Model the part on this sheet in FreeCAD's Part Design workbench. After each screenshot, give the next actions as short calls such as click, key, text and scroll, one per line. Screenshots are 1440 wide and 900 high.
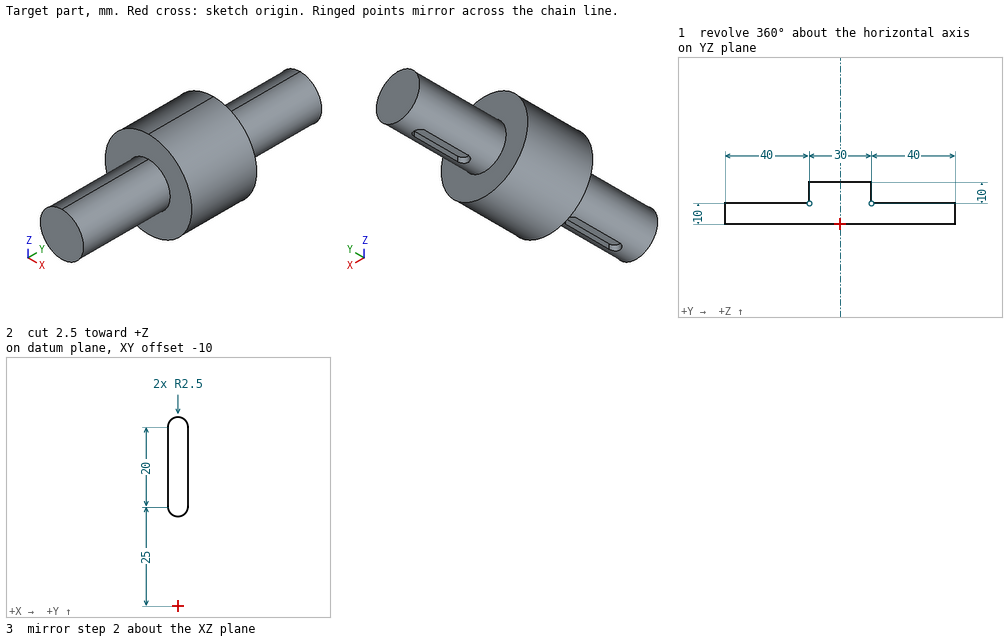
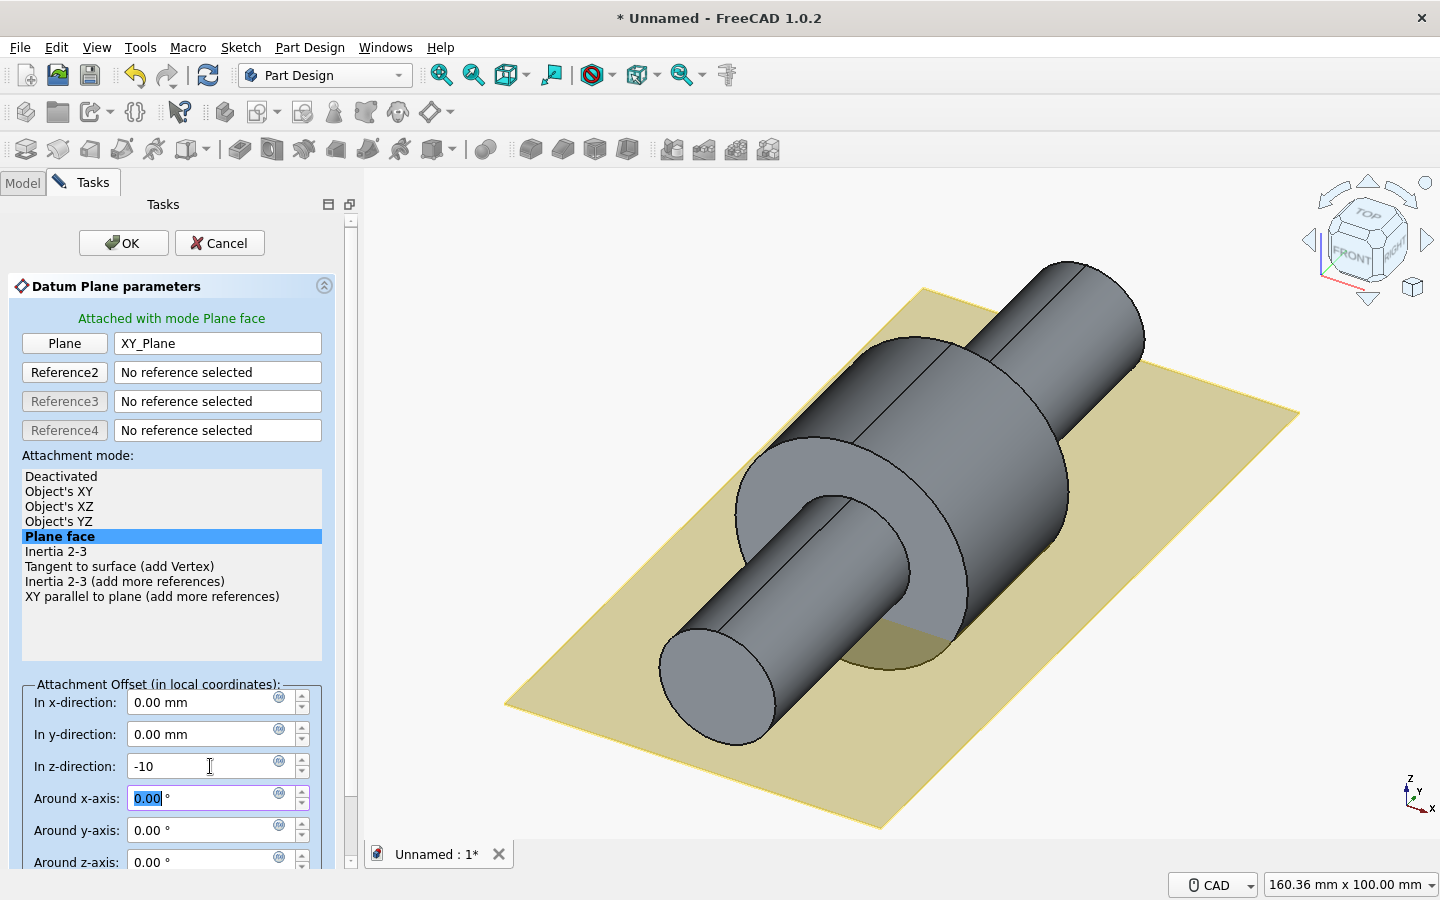
click(124, 243)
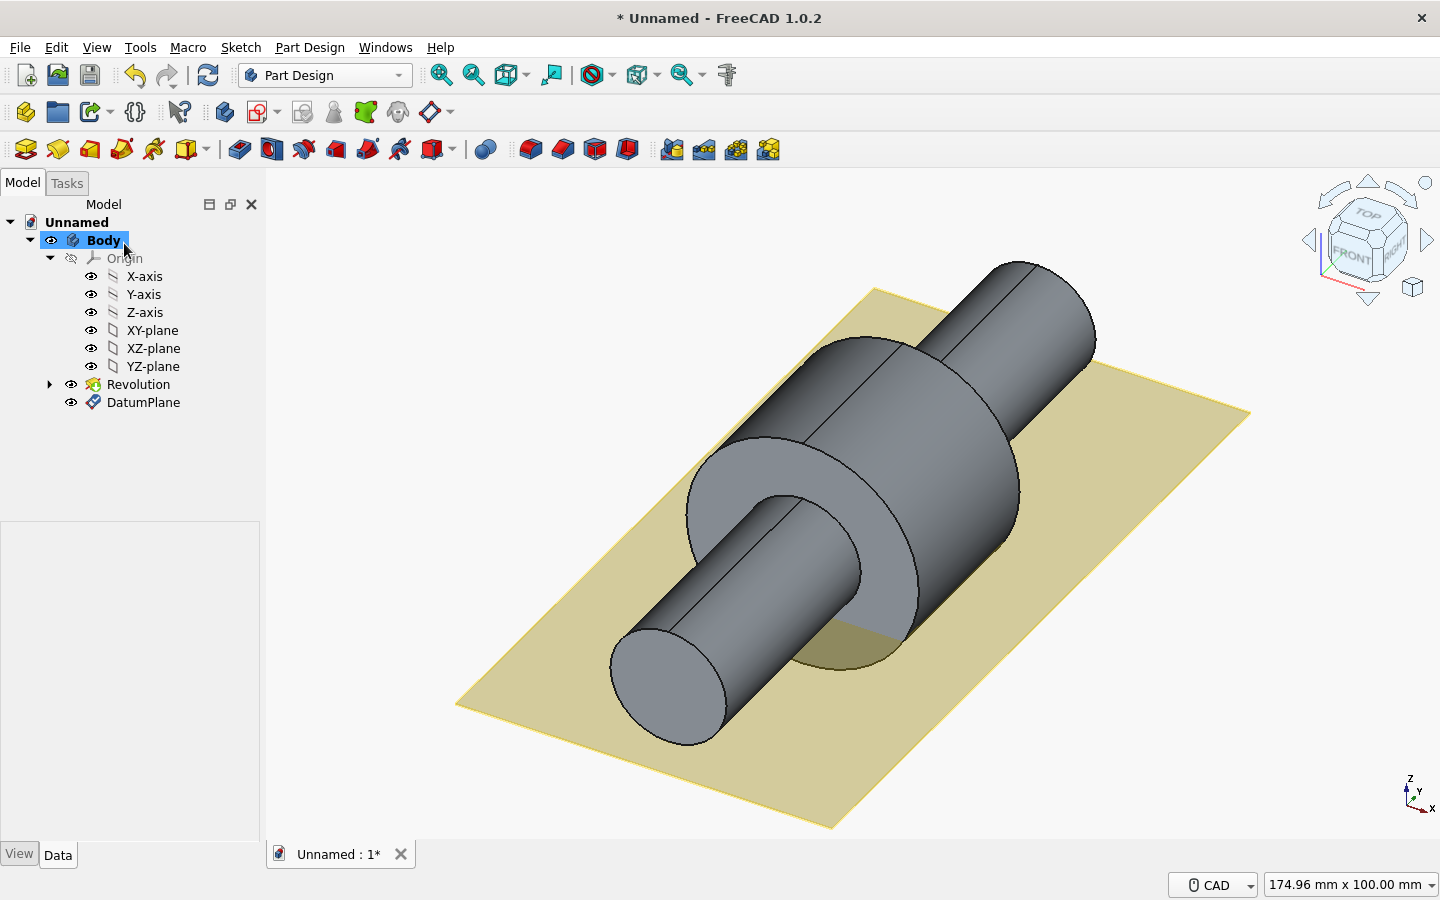
click(116, 402)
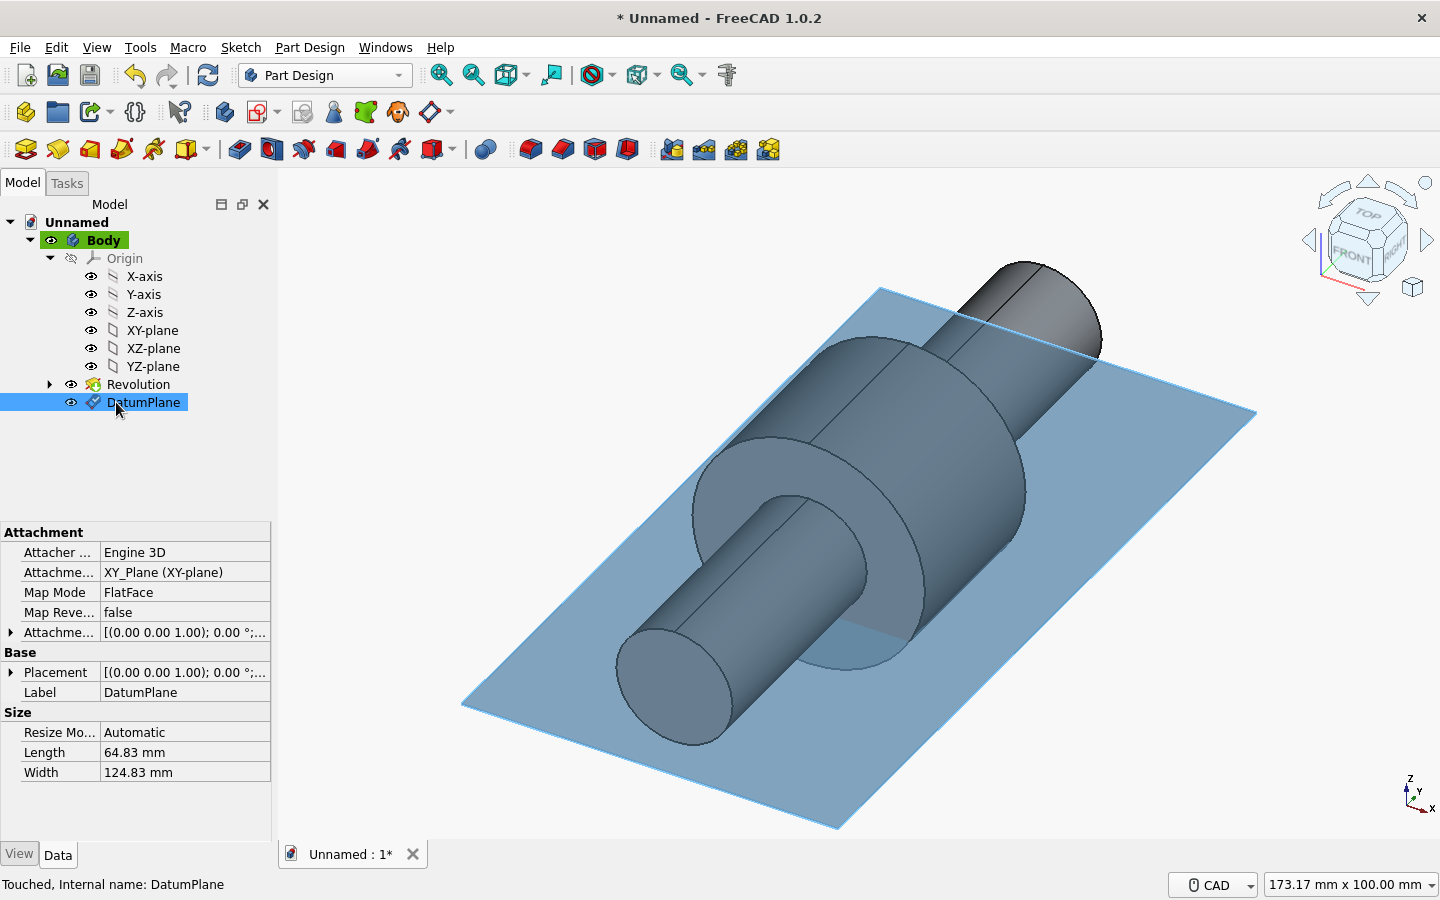
click(258, 112)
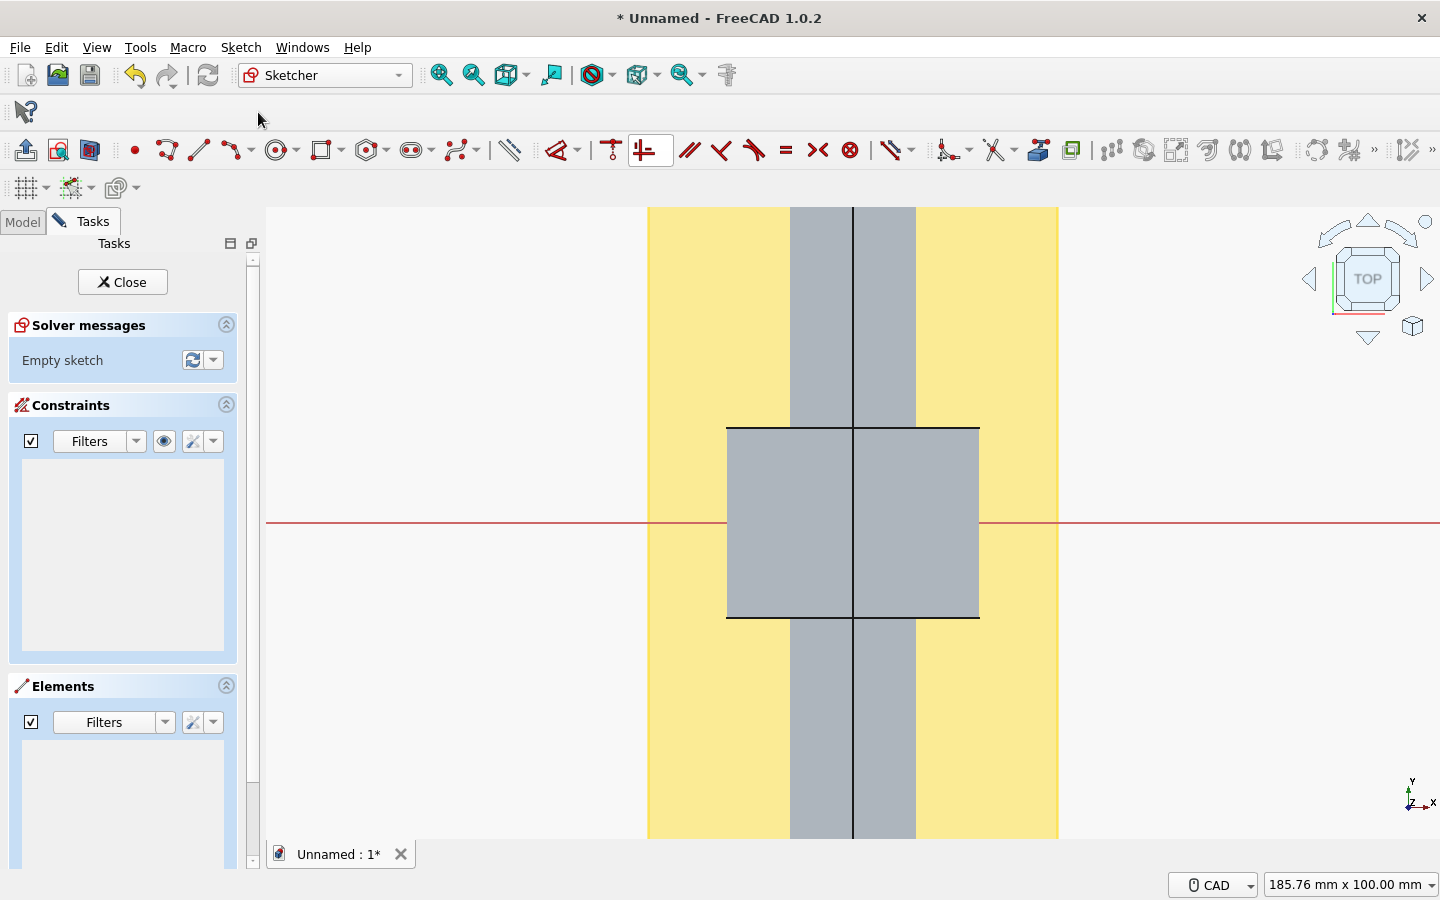
click(90, 150)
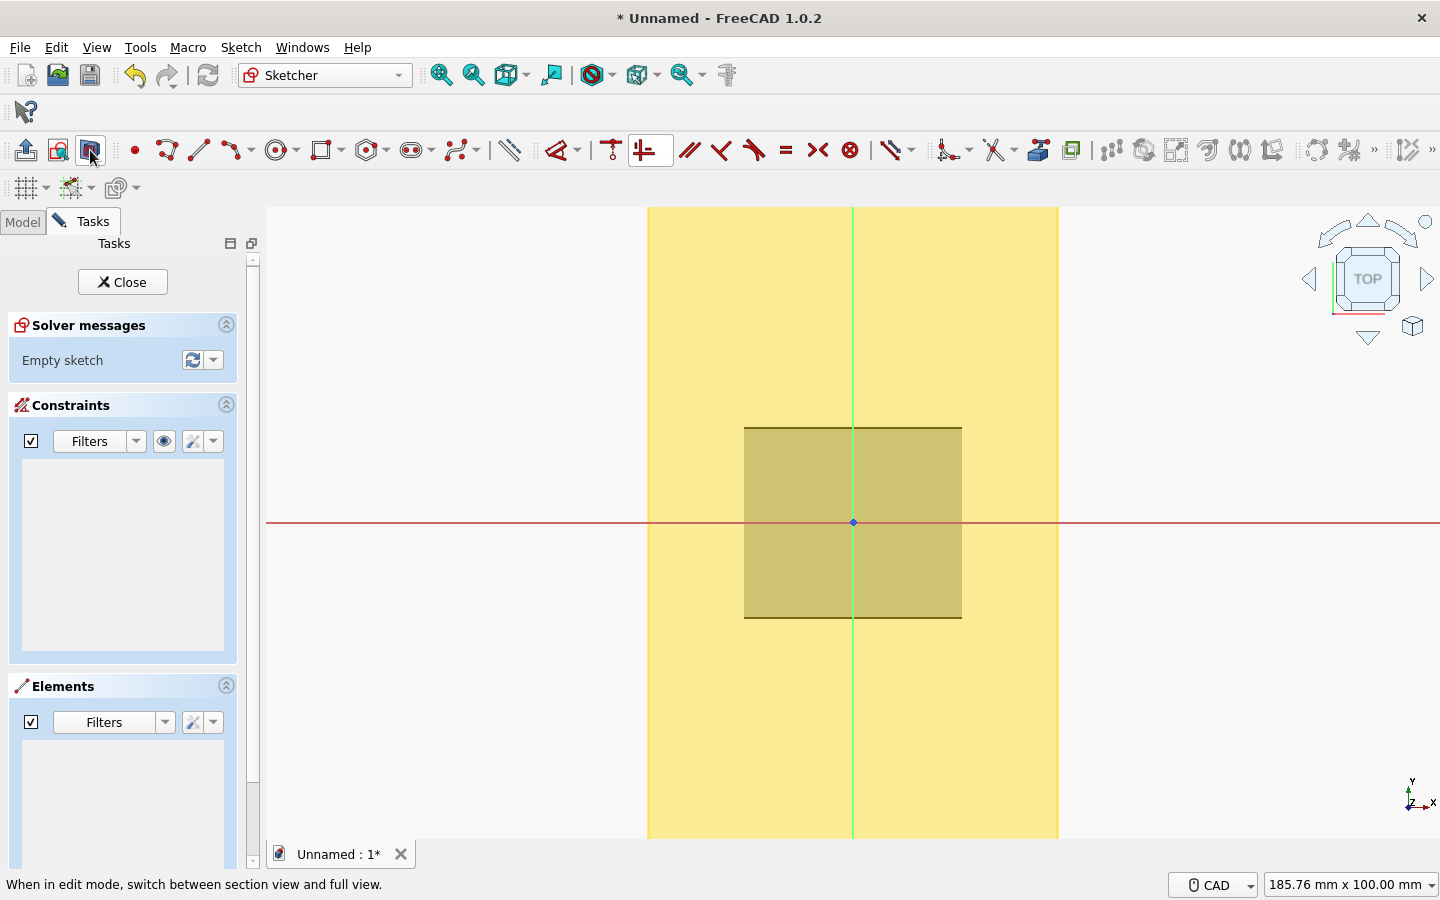
scroll(475, 811, down, 1)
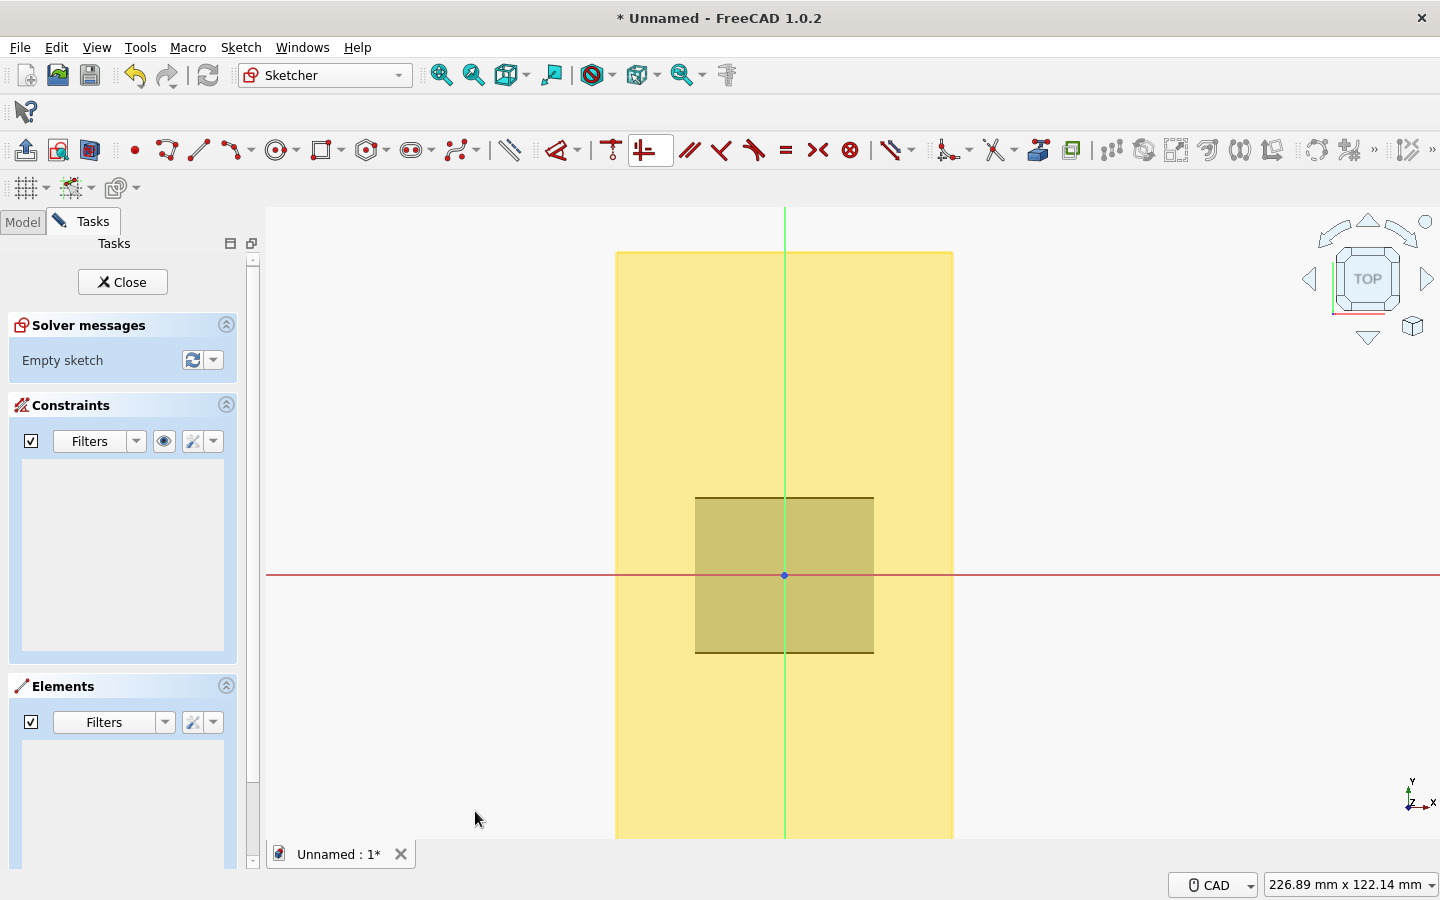
scroll(785, 367, up, 3)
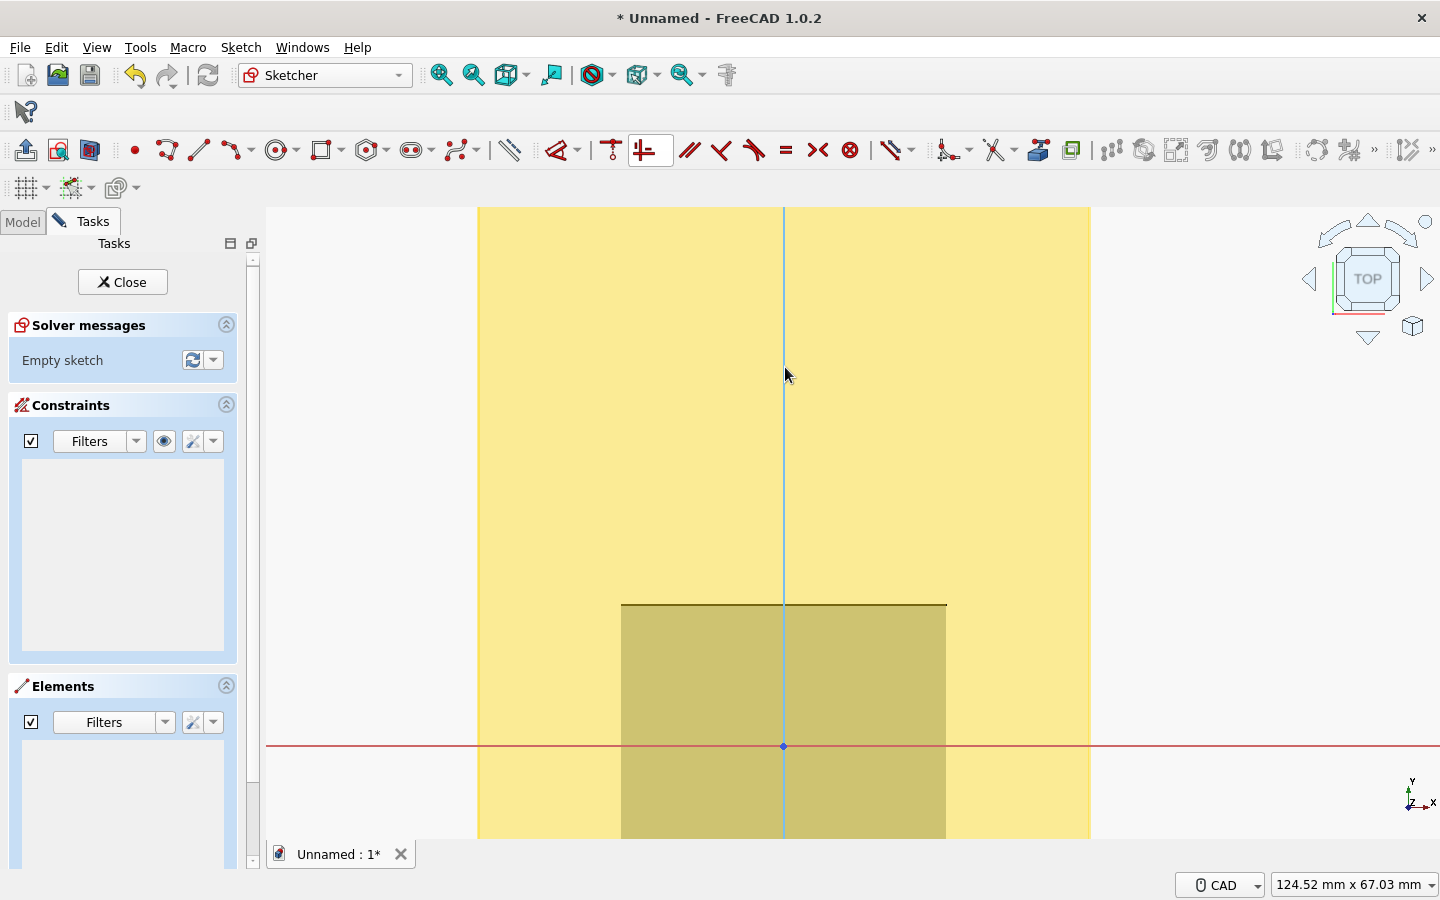
click(412, 150)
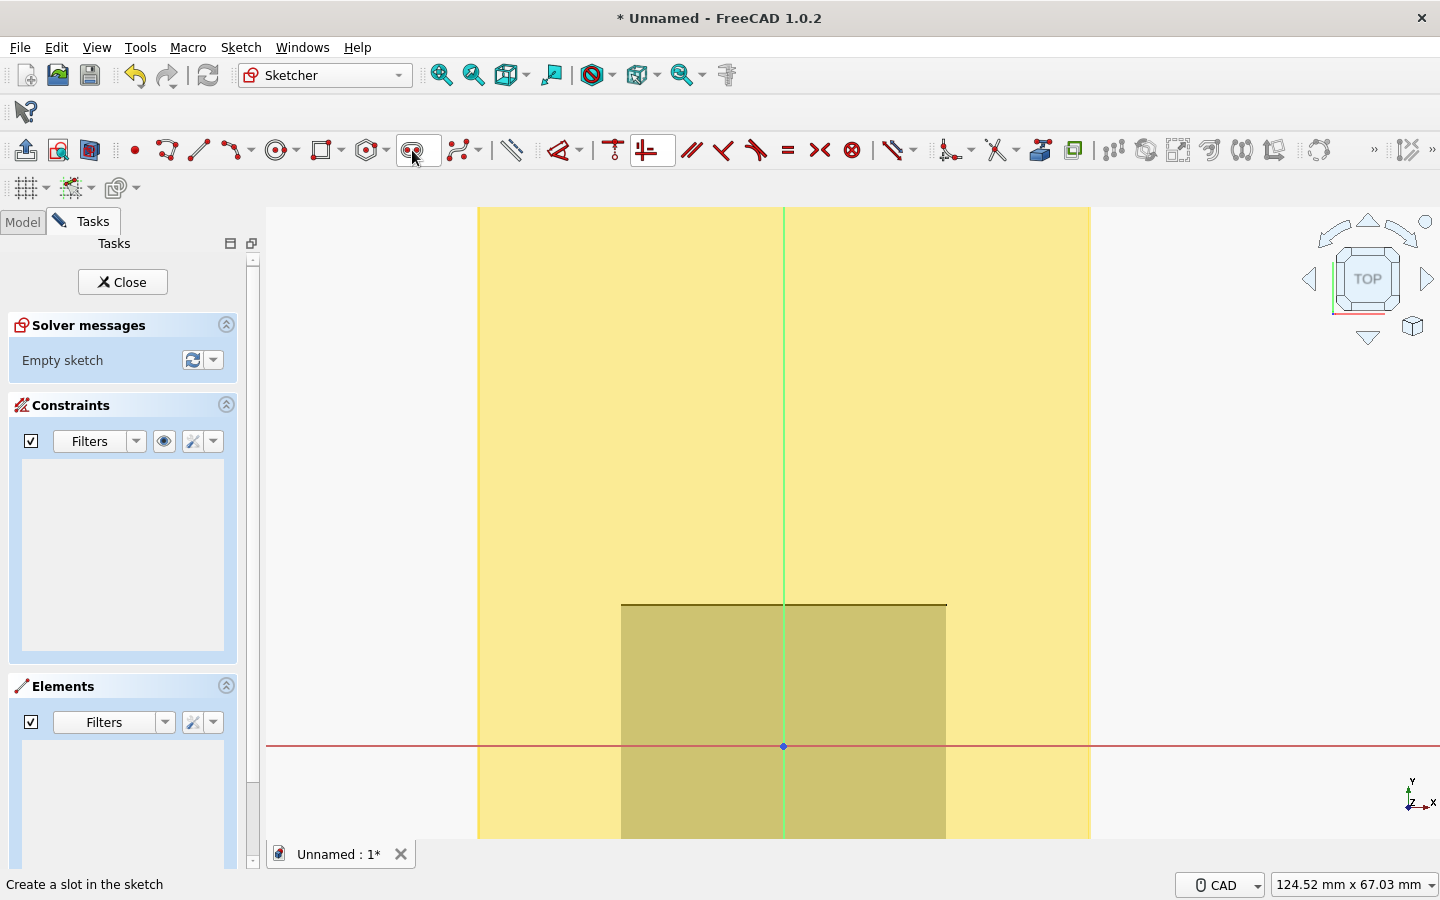
click(784, 511)